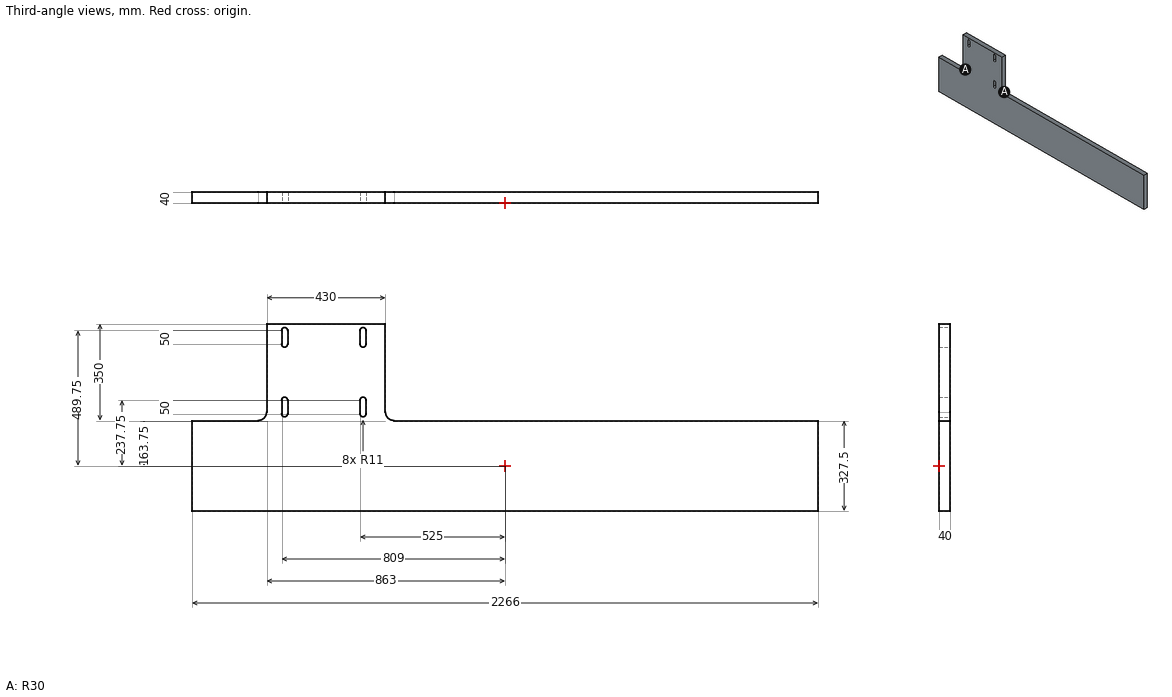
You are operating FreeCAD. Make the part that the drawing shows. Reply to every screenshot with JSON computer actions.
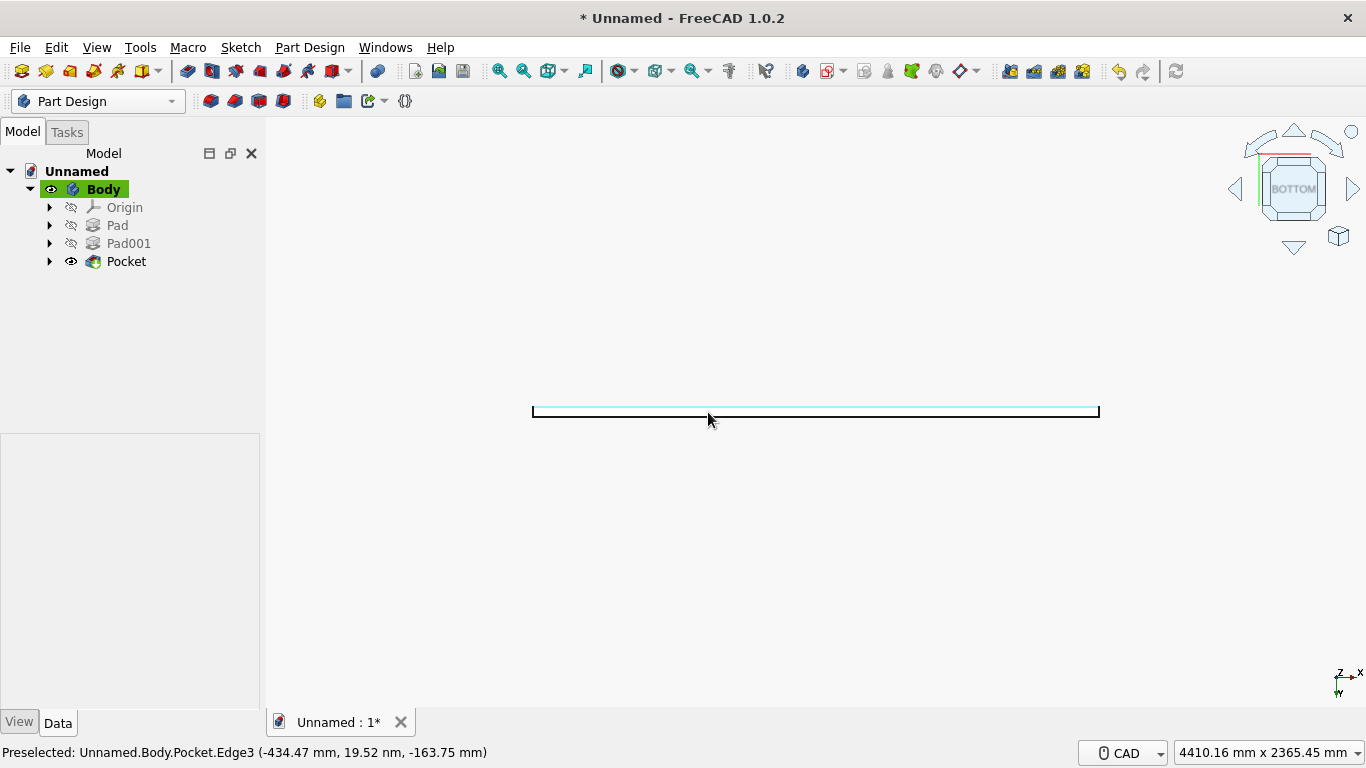
{"action": "key", "text": "4"}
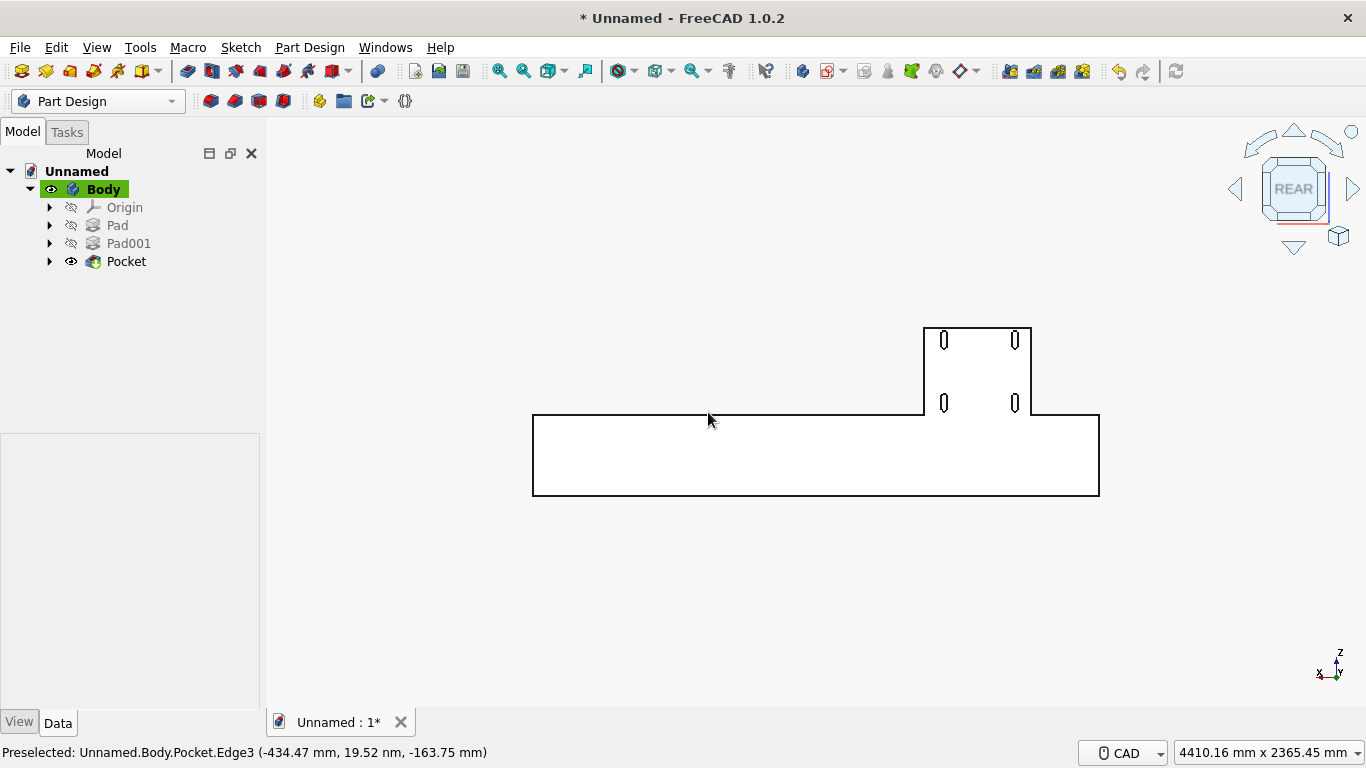
{"action": "scroll", "coordinate": [924, 414], "scroll_direction": "up", "scroll_amount": 7}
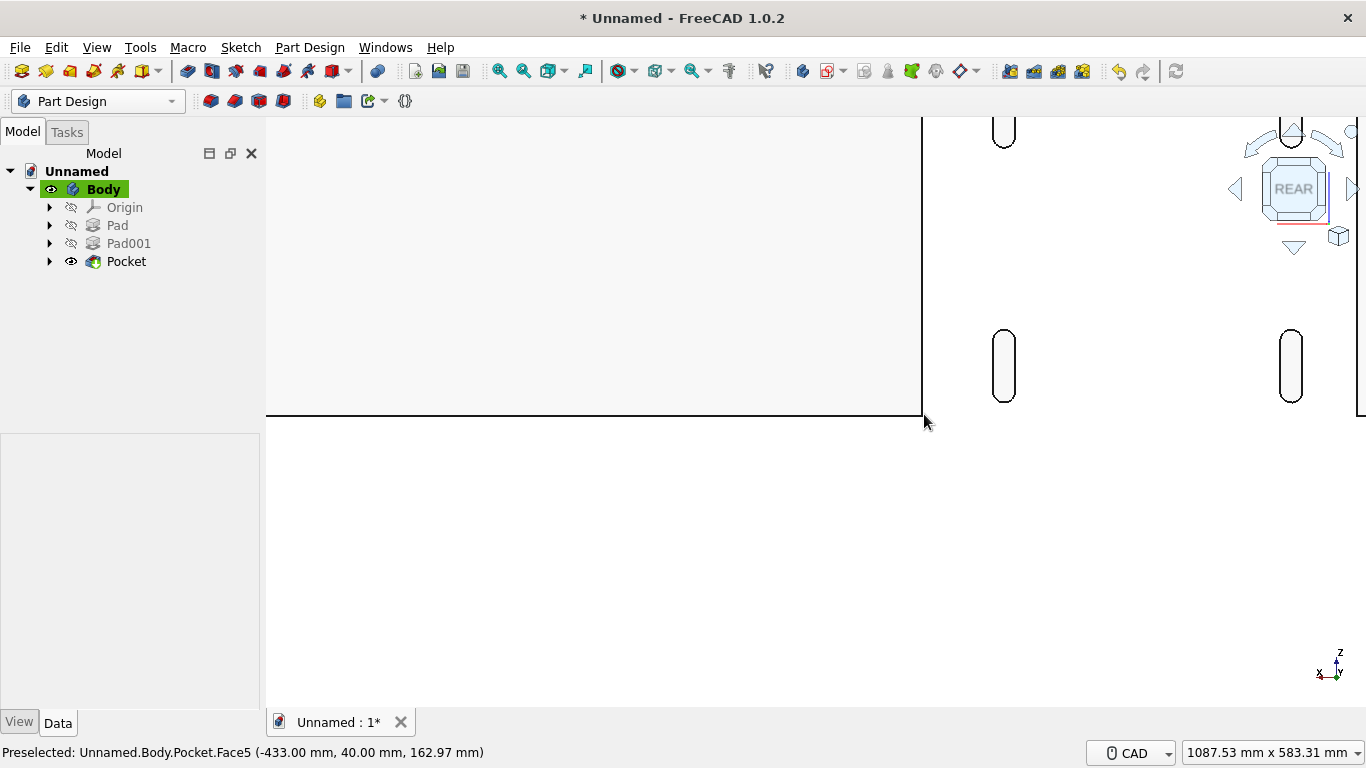
{"action": "left_click", "coordinate": [500, 72]}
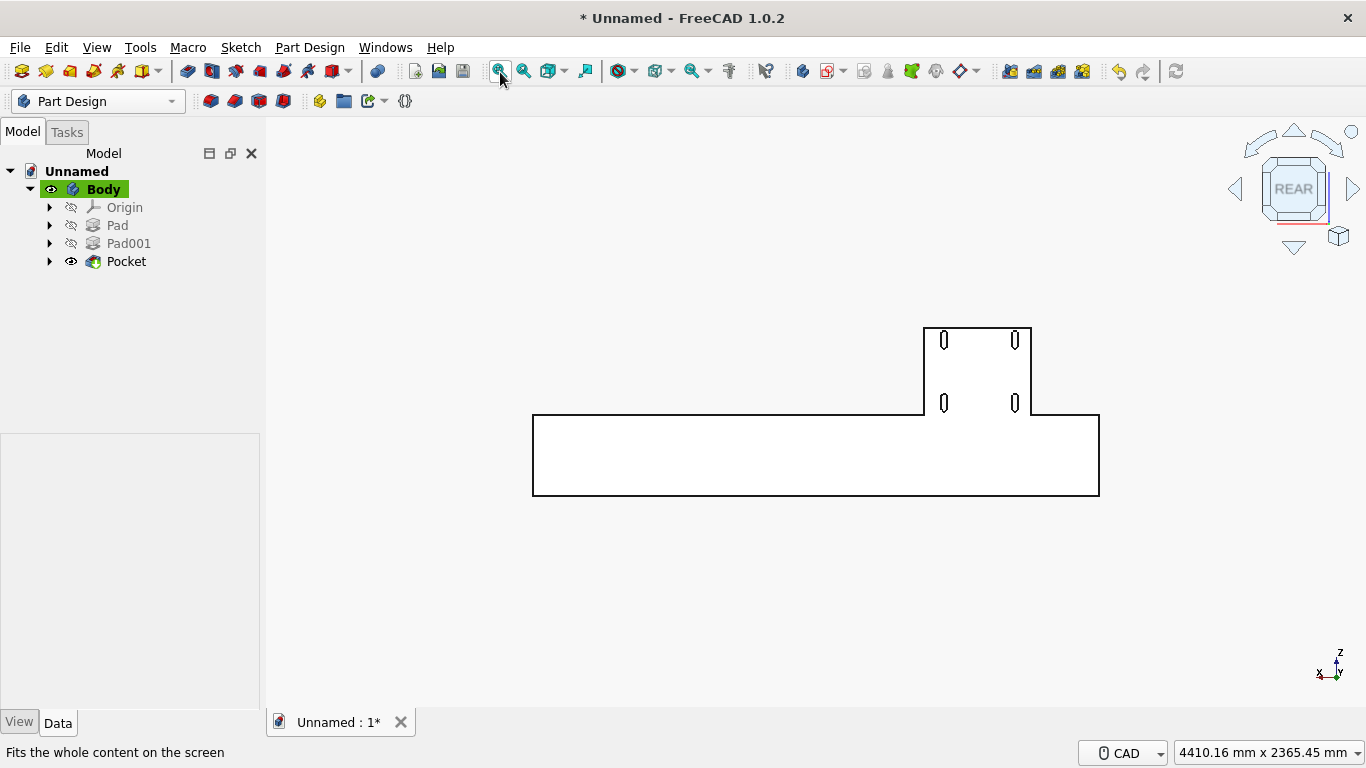
{"action": "key", "text": "6"}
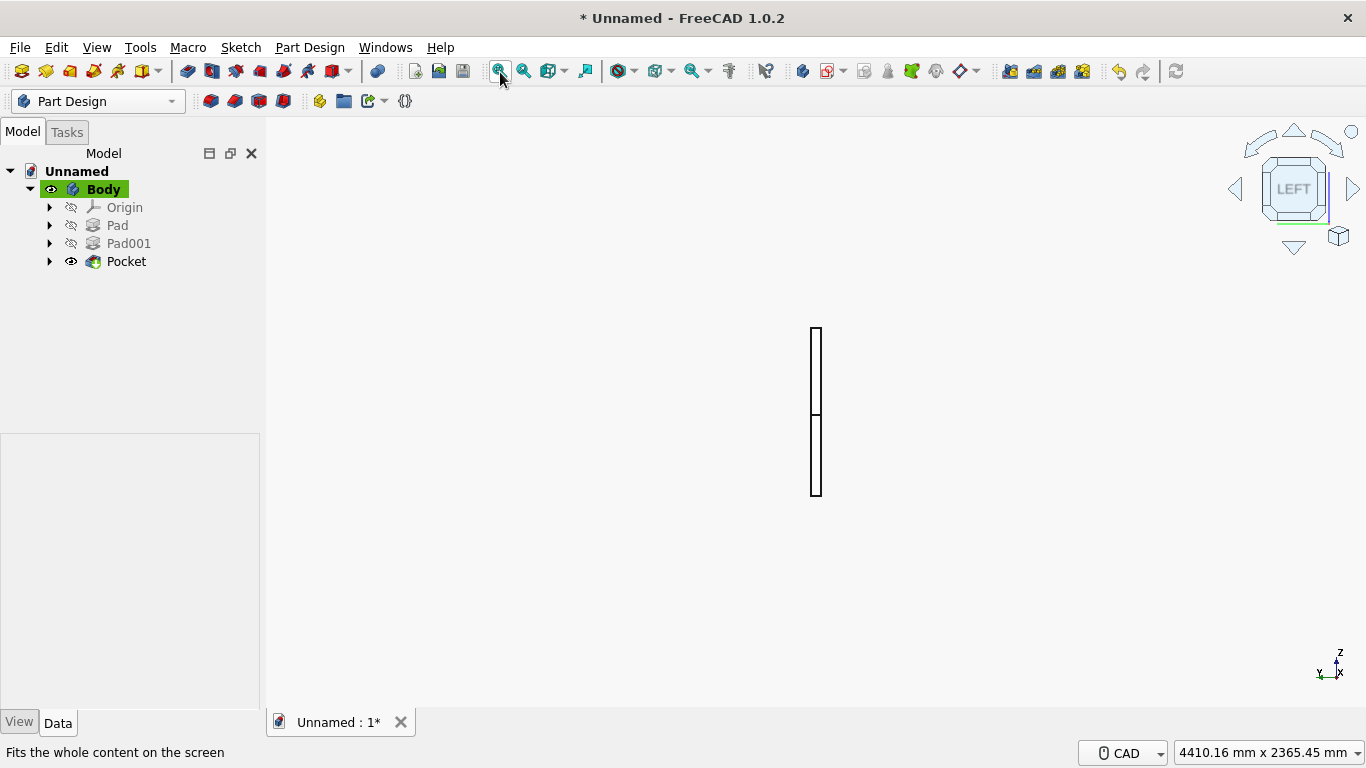
{"action": "left_click", "coordinate": [500, 72]}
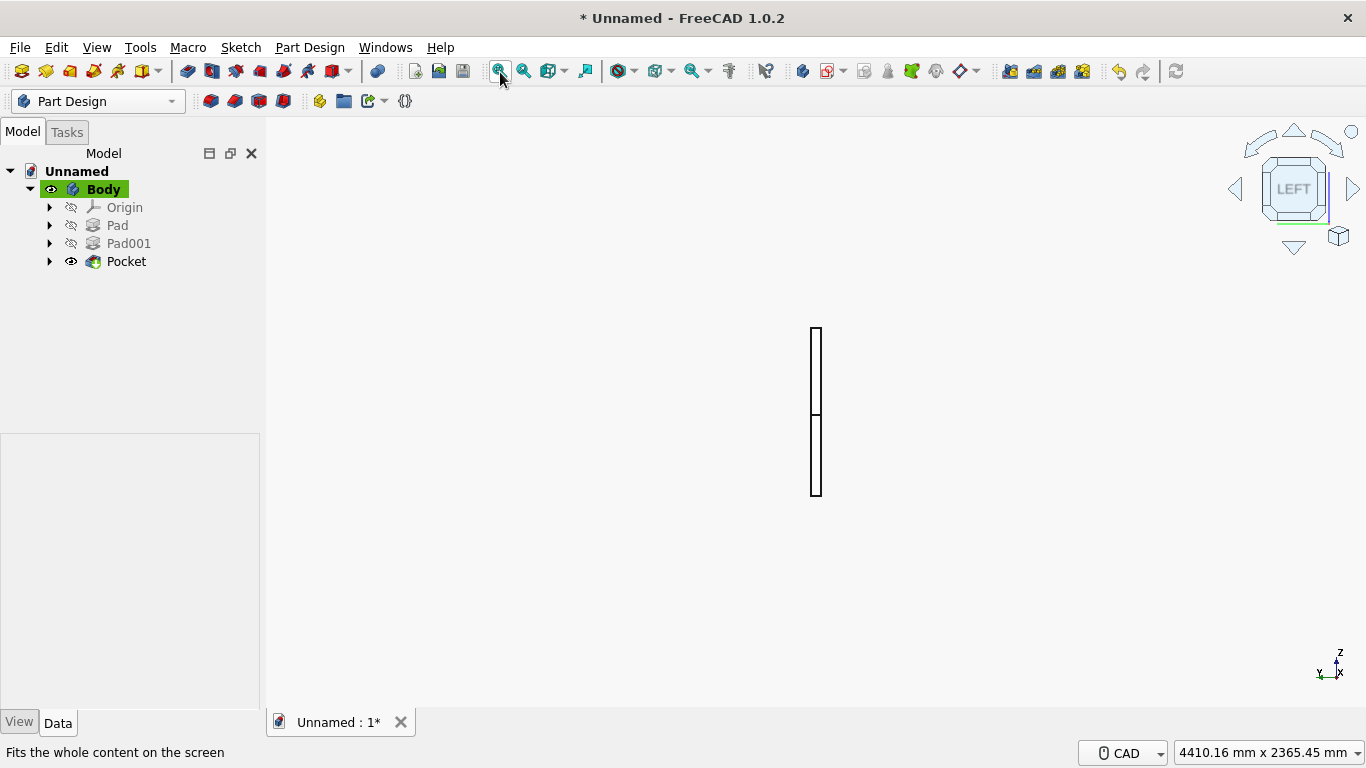
{"action": "scroll", "coordinate": [816, 414], "scroll_direction": "up", "scroll_amount": 7}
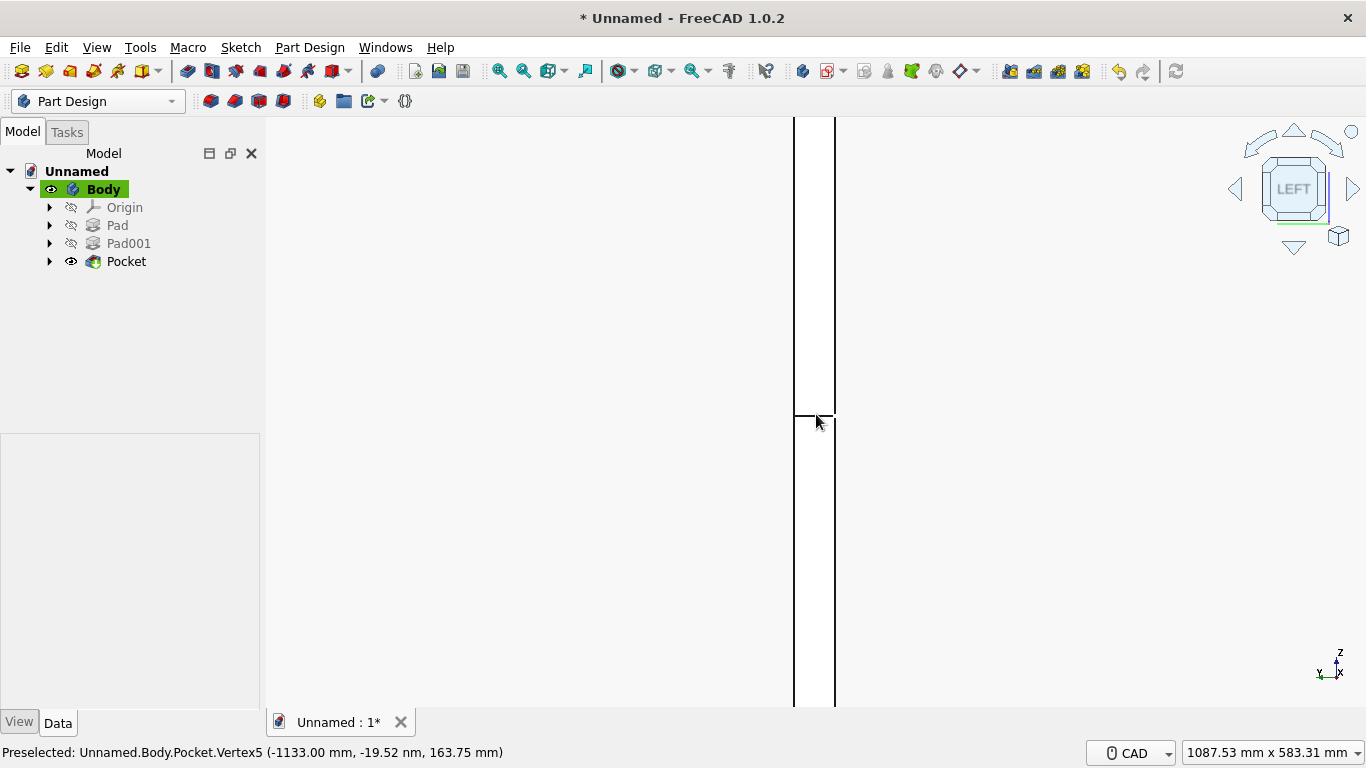
{"action": "key", "text": "v f"}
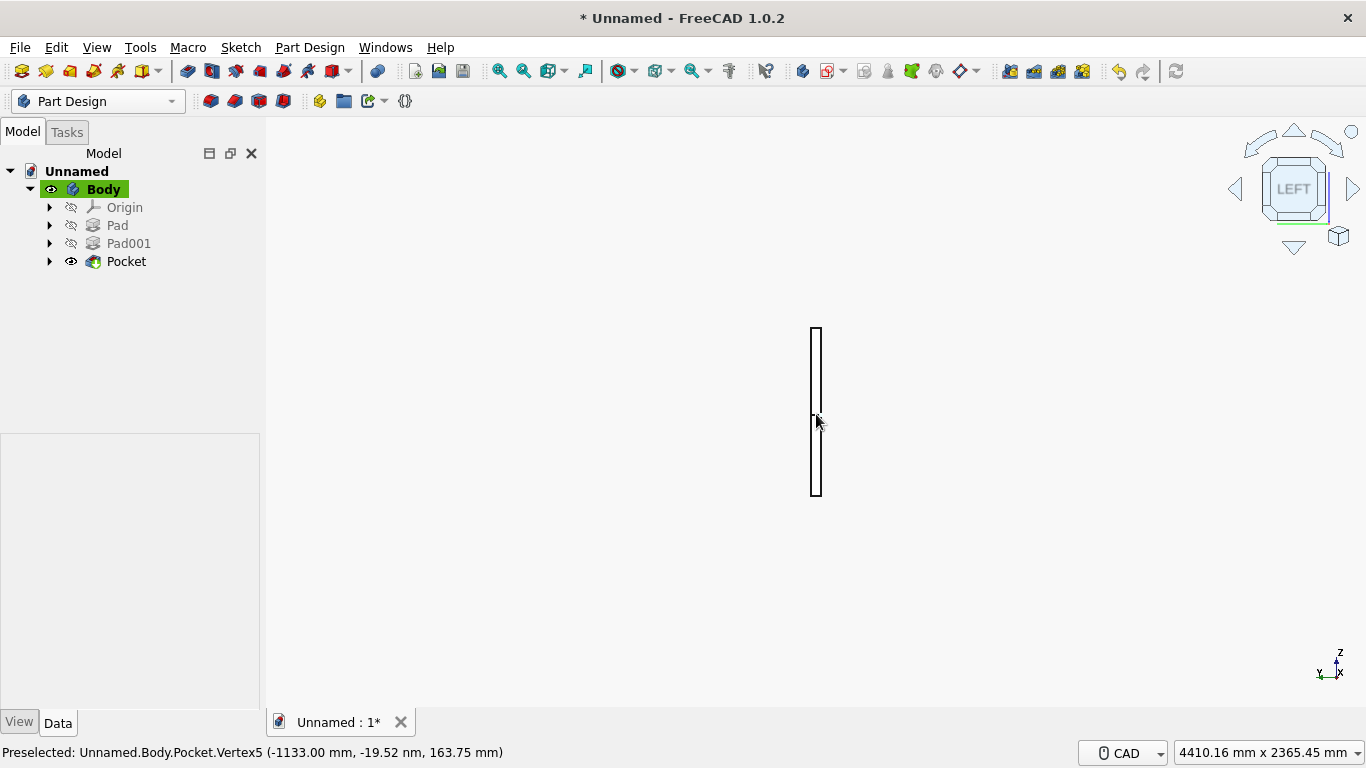
{"action": "key", "text": "v 3"}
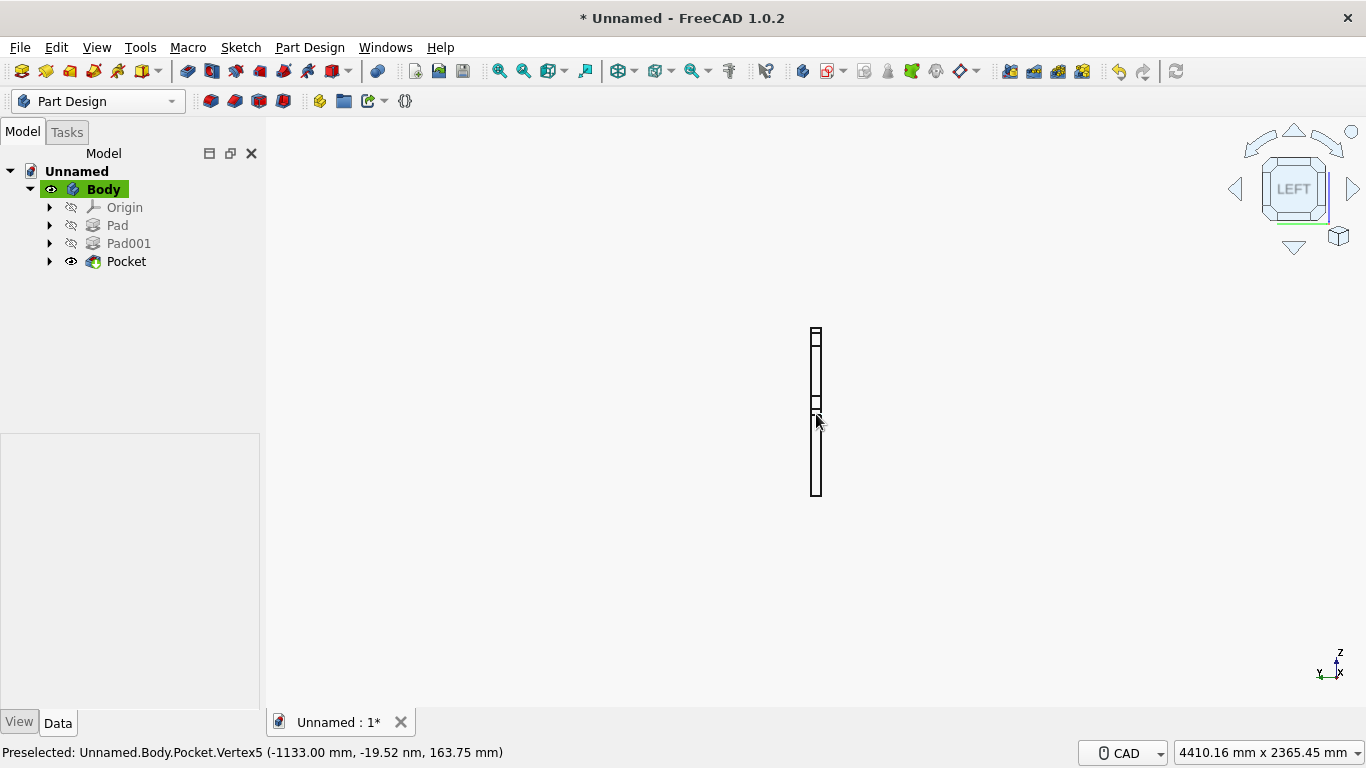
{"action": "key", "text": "0"}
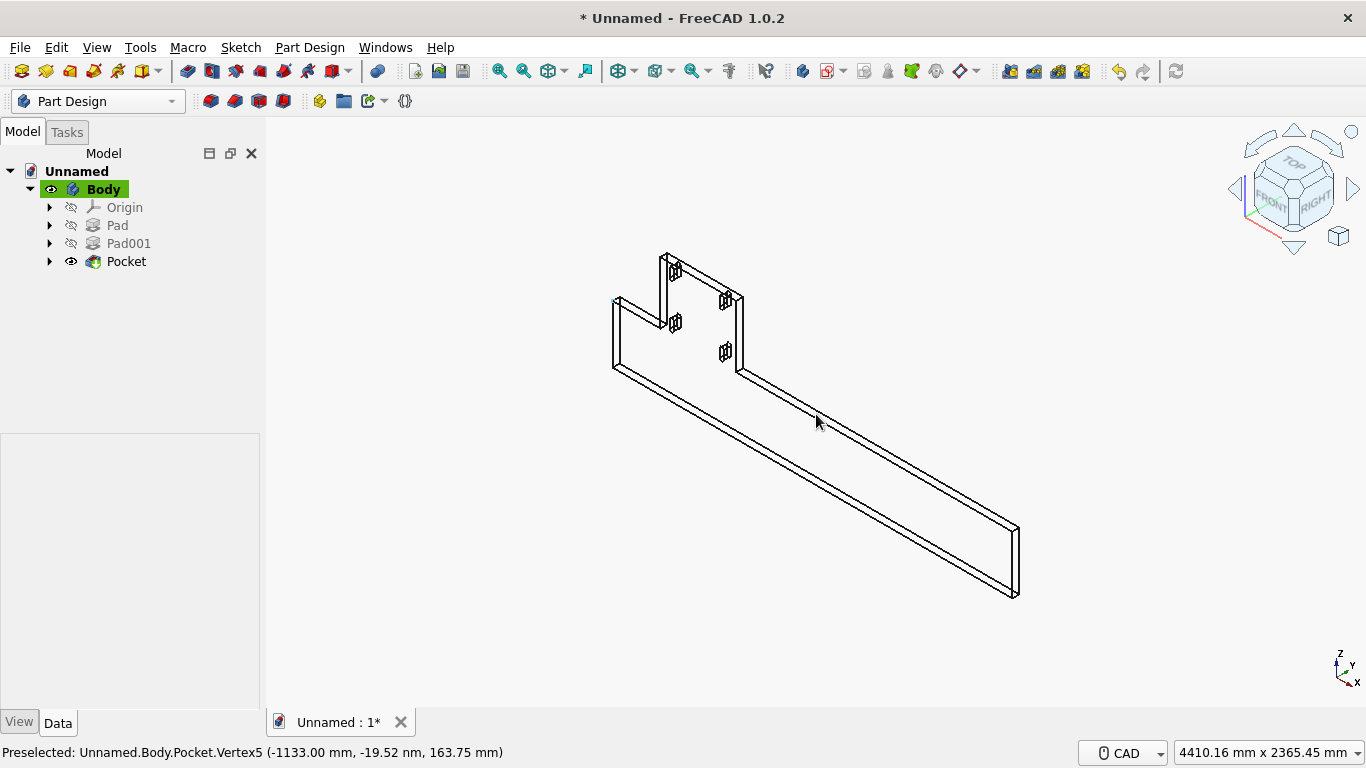
{"action": "scroll", "coordinate": [740, 369], "scroll_direction": "up", "scroll_amount": 7}